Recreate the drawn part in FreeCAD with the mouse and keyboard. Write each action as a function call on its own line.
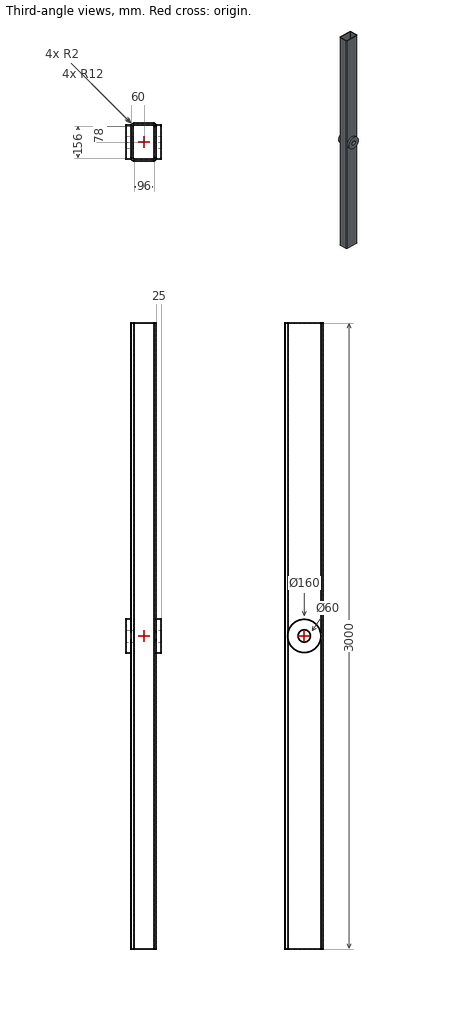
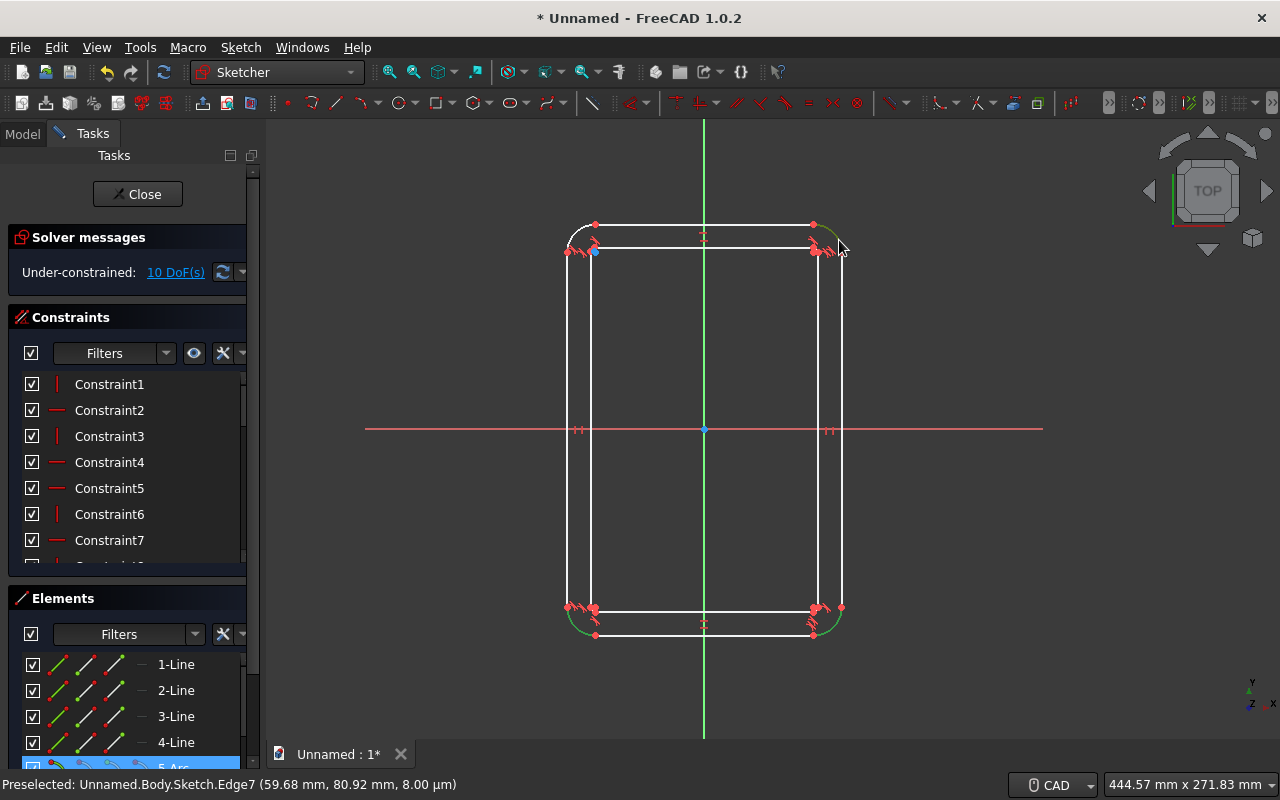
click(583, 228)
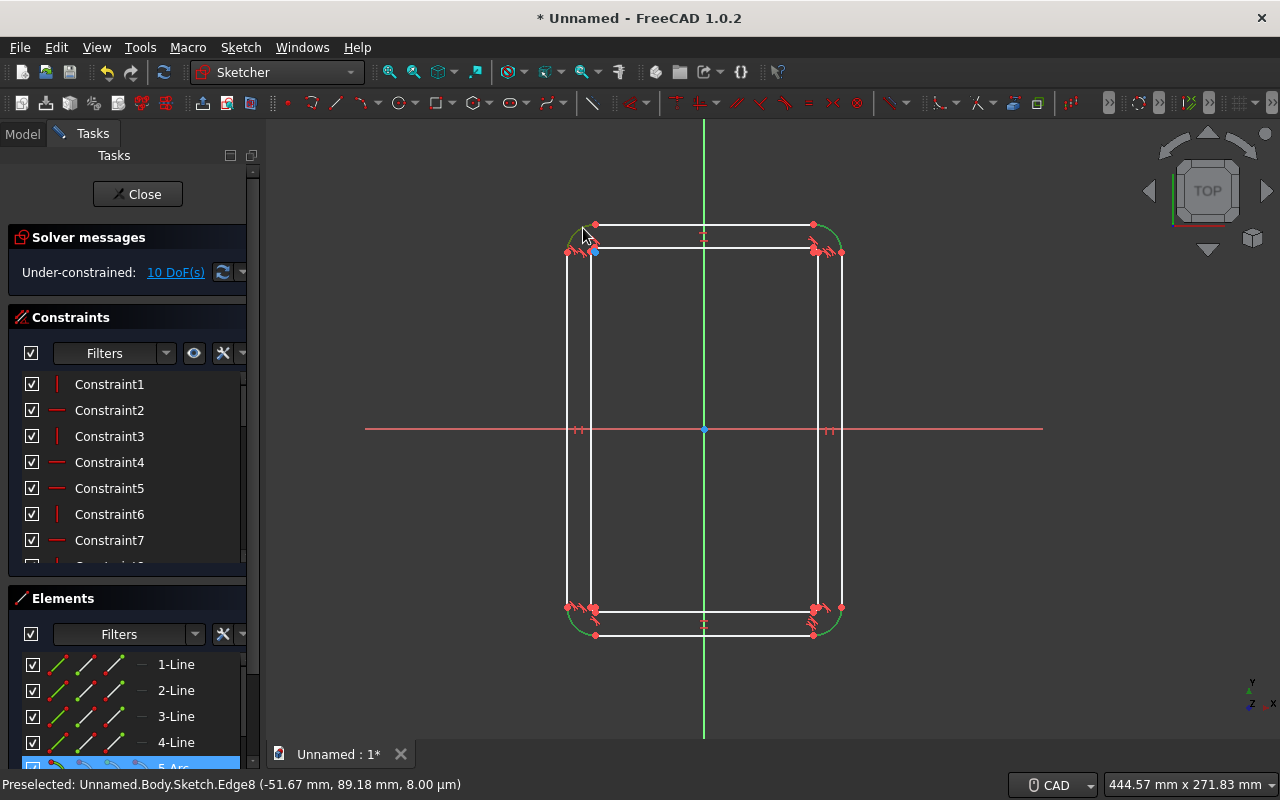
click(810, 104)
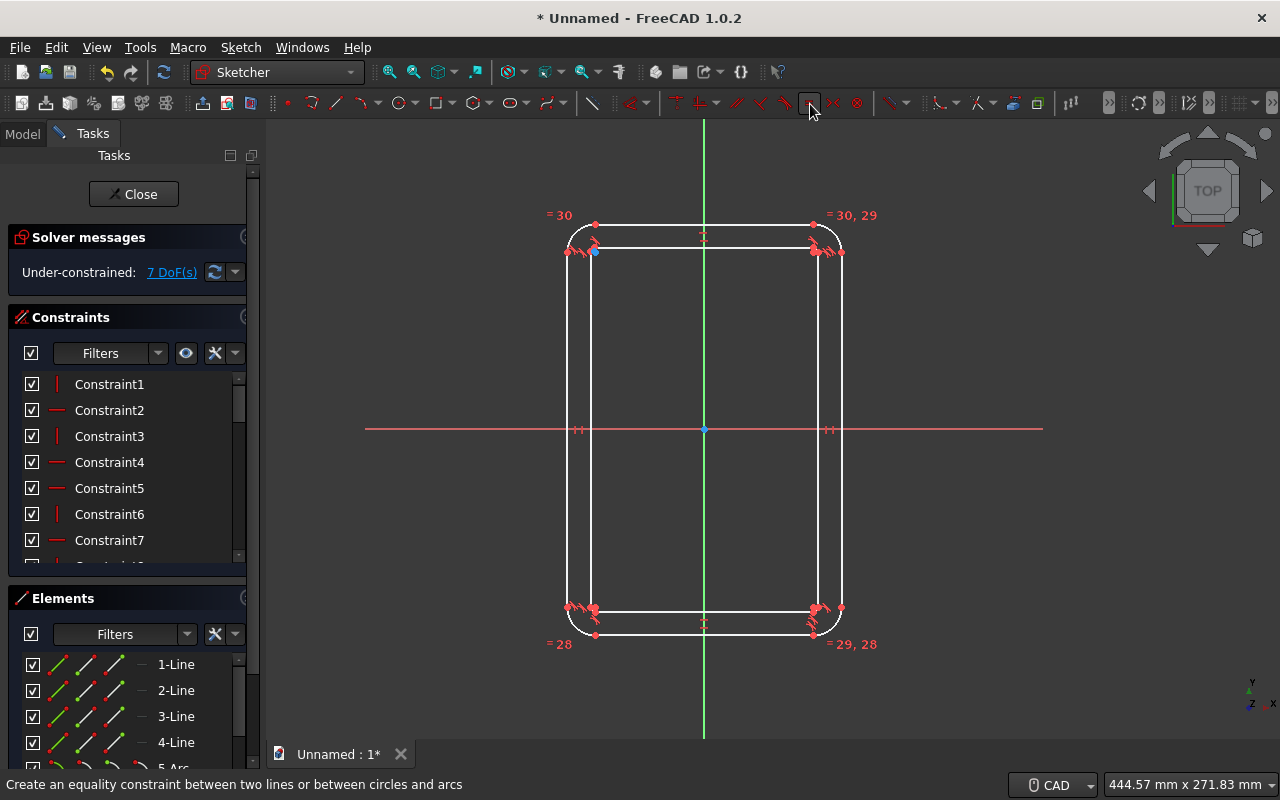
scroll(817, 249, up, 7)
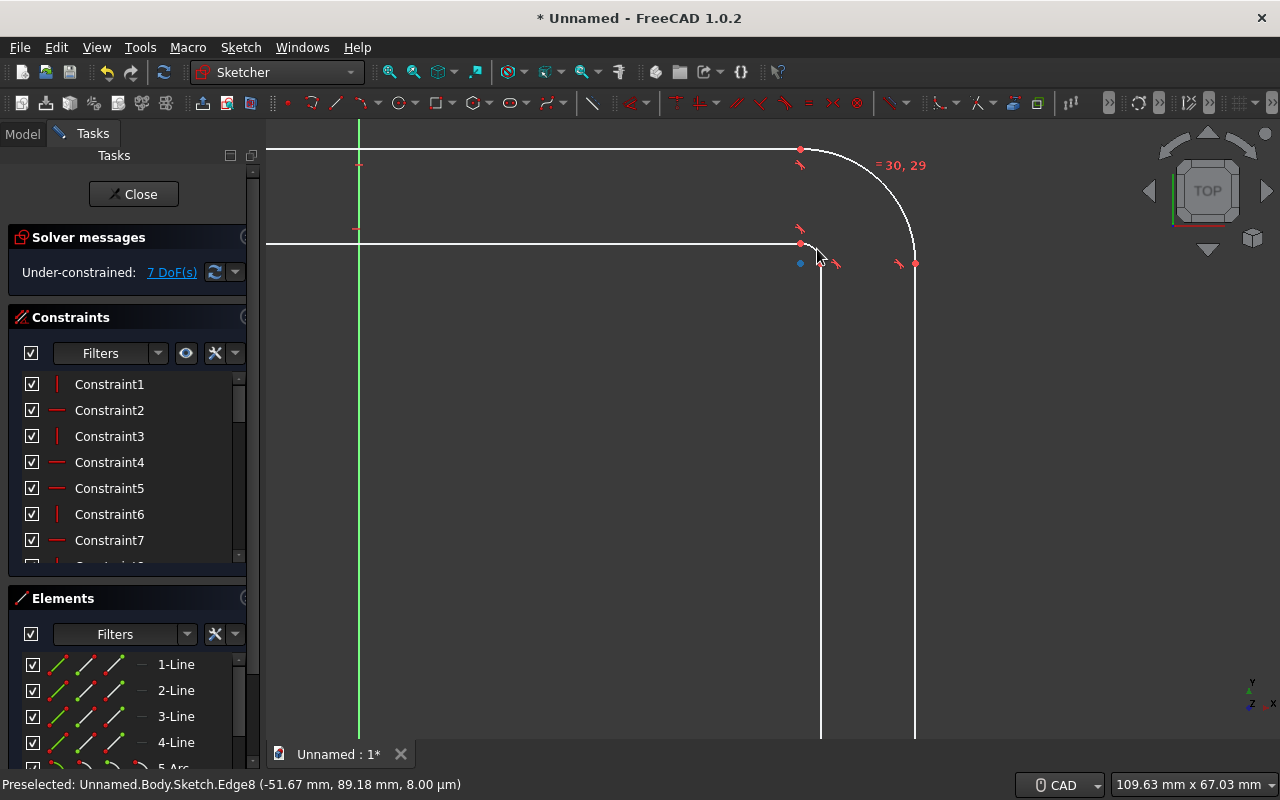
click(815, 249)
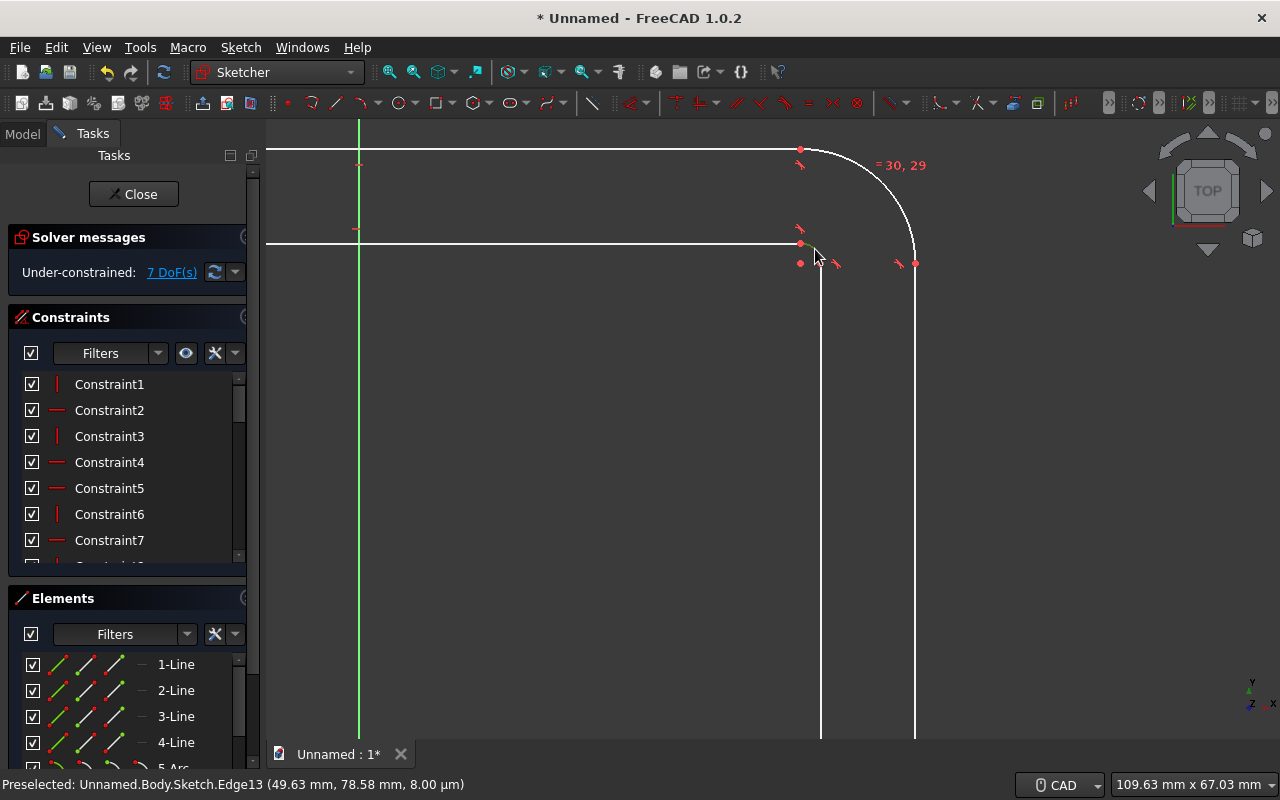
scroll(818, 249, down, 7)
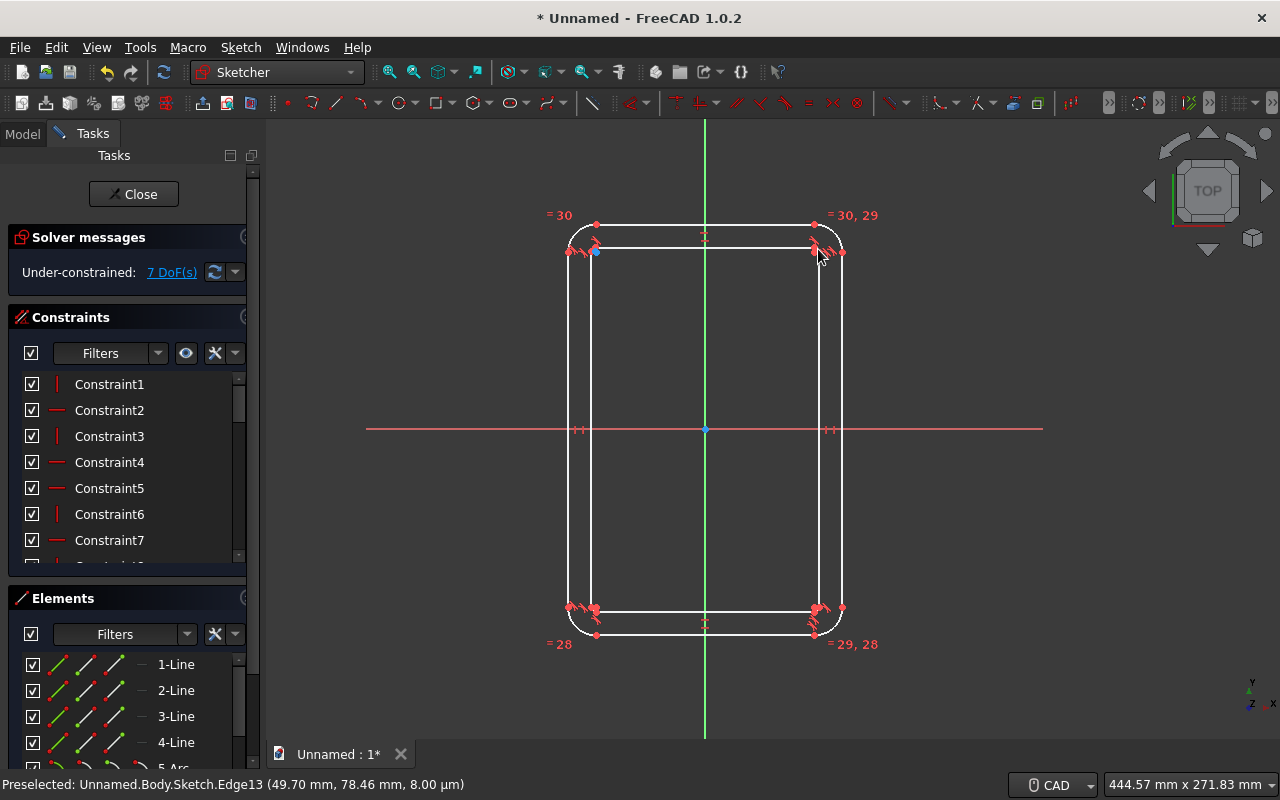
scroll(592, 249, up, 8)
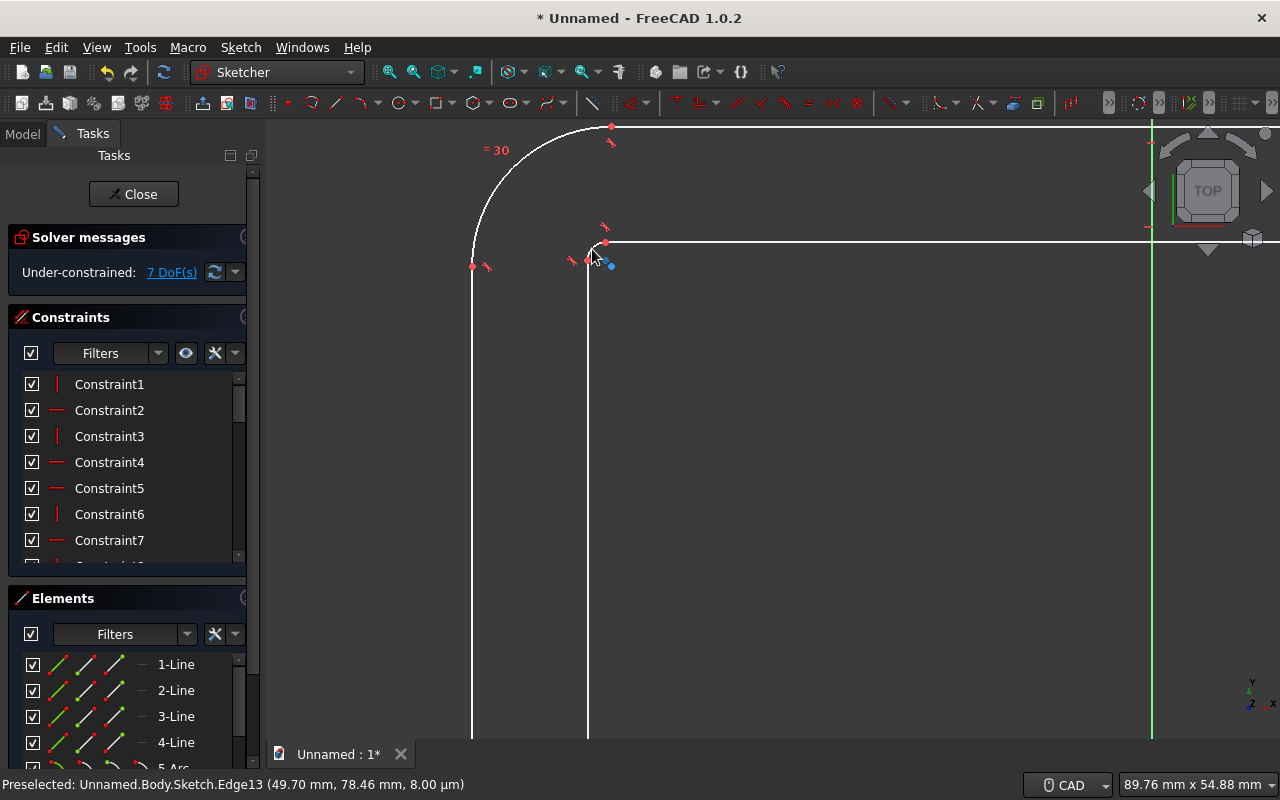
click(593, 248)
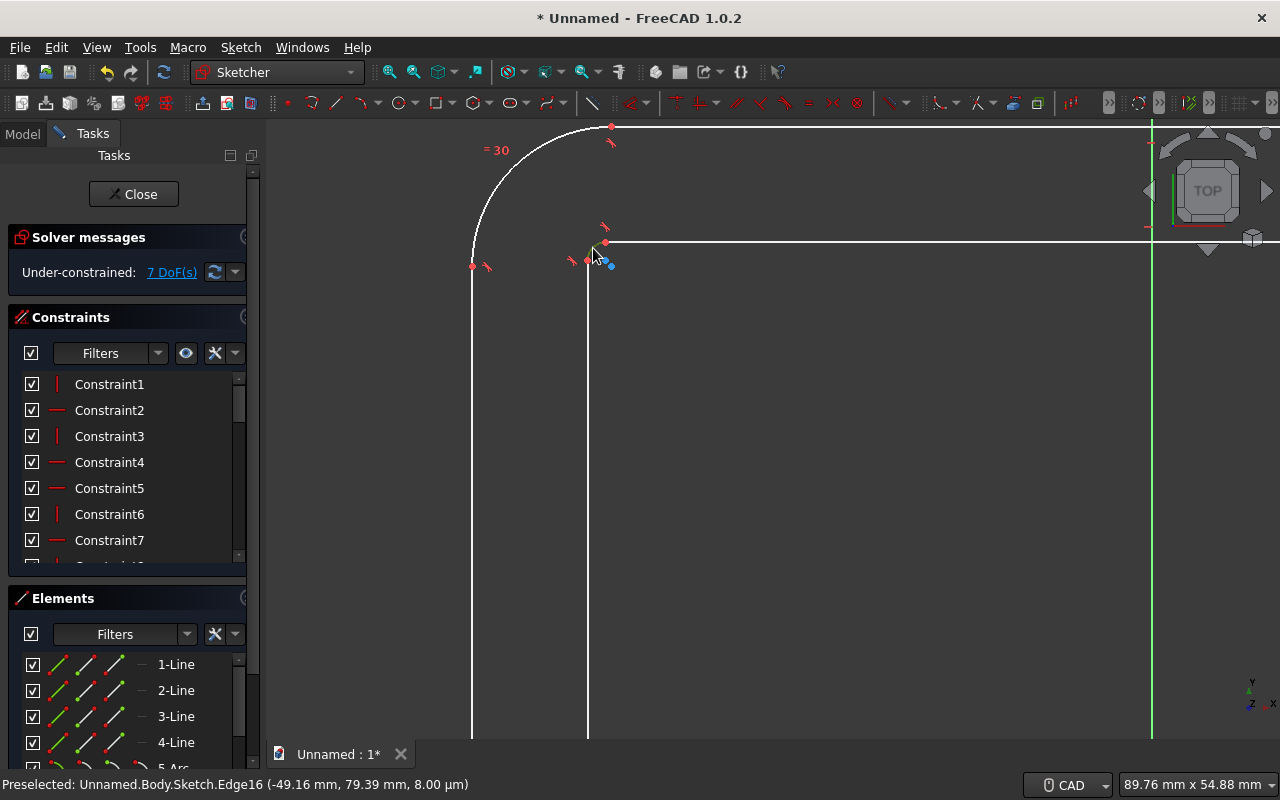
click(810, 104)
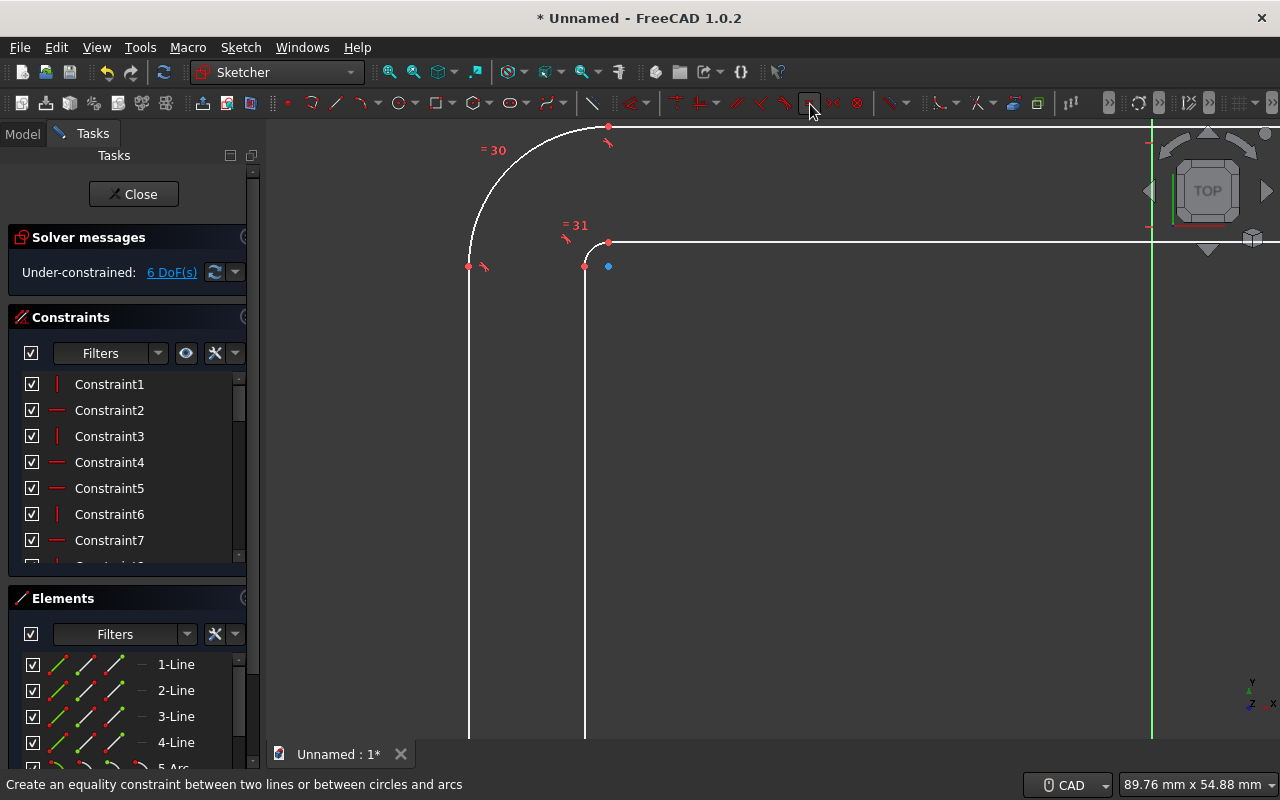
click(630, 104)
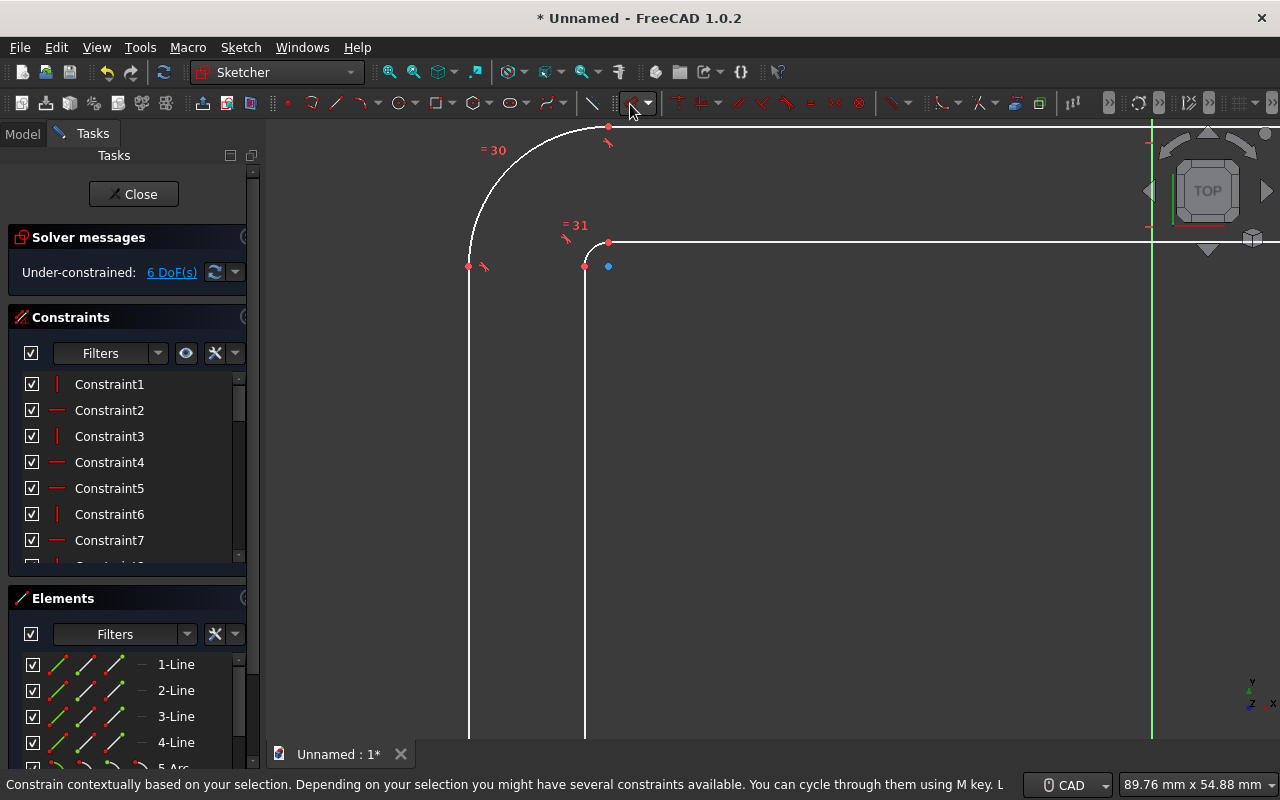
scroll(591, 249, down, 8)